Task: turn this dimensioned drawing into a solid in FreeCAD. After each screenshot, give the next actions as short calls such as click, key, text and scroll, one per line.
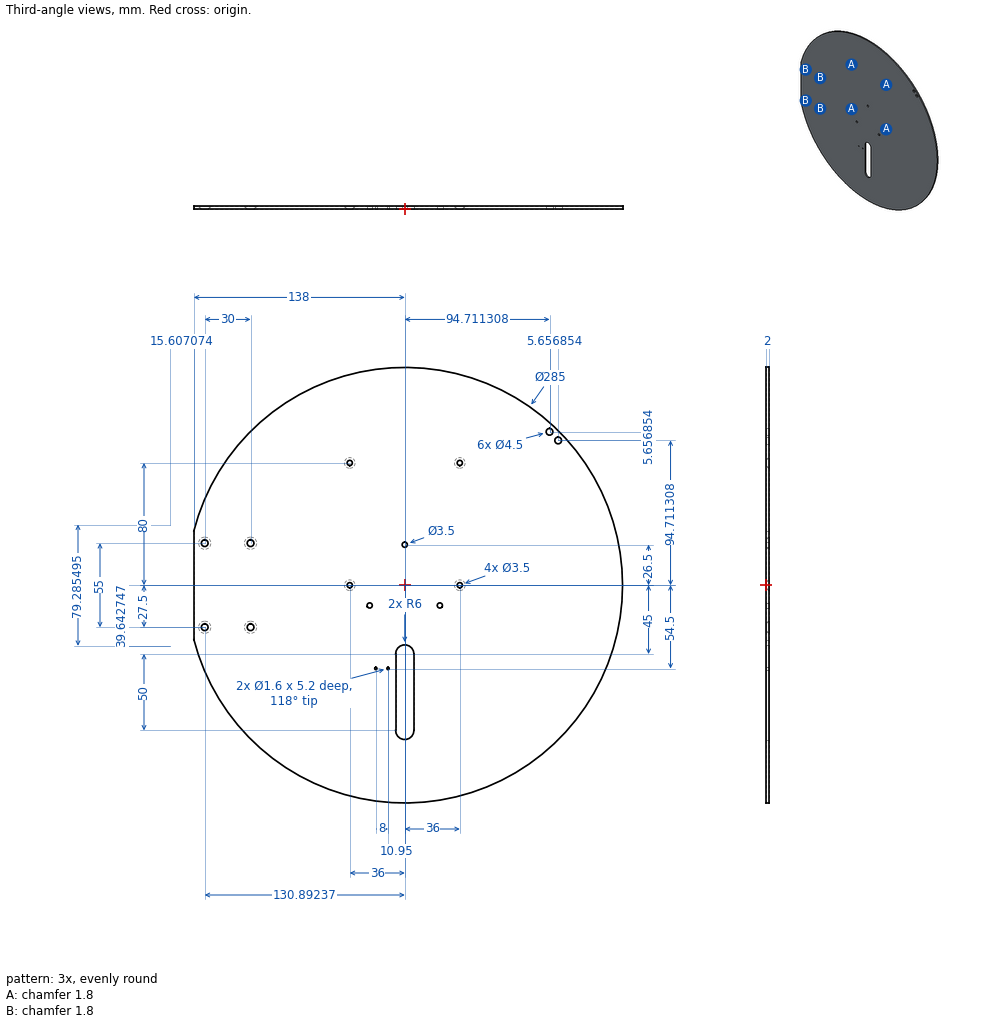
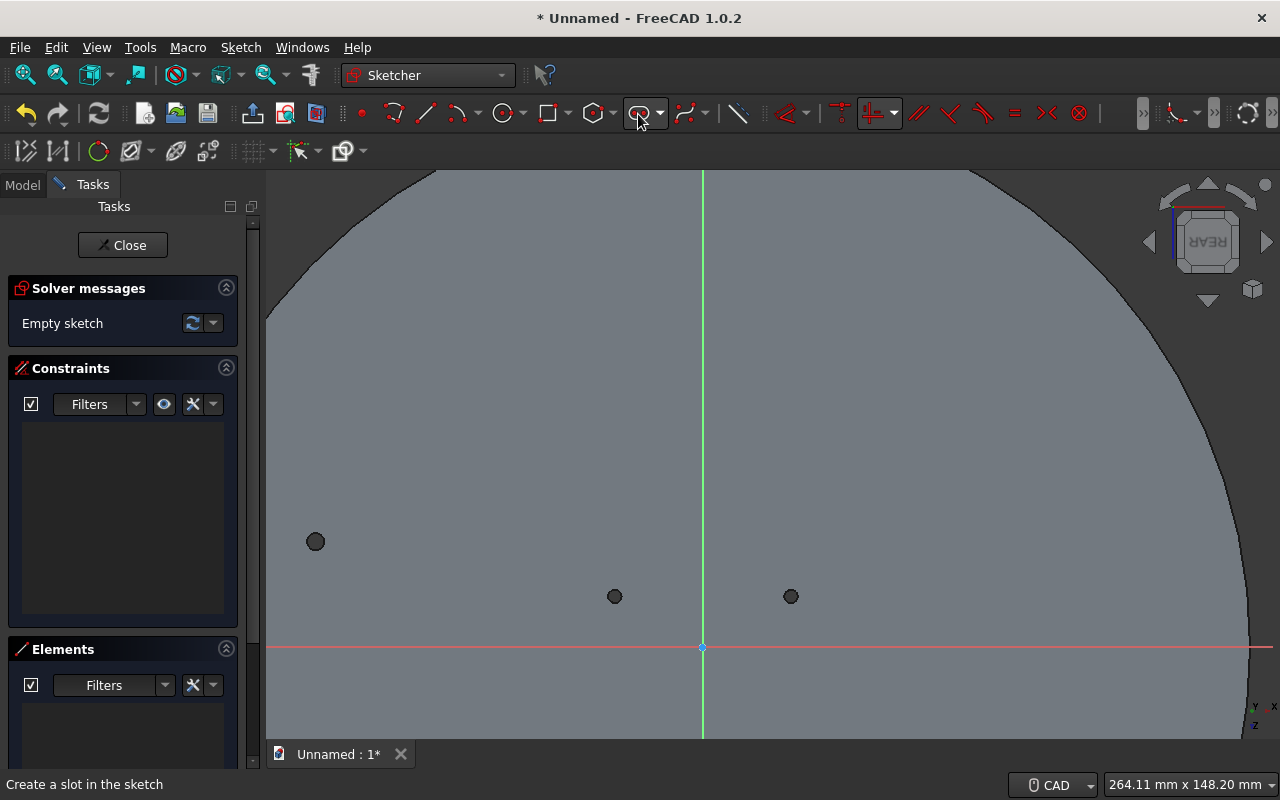
click(703, 475)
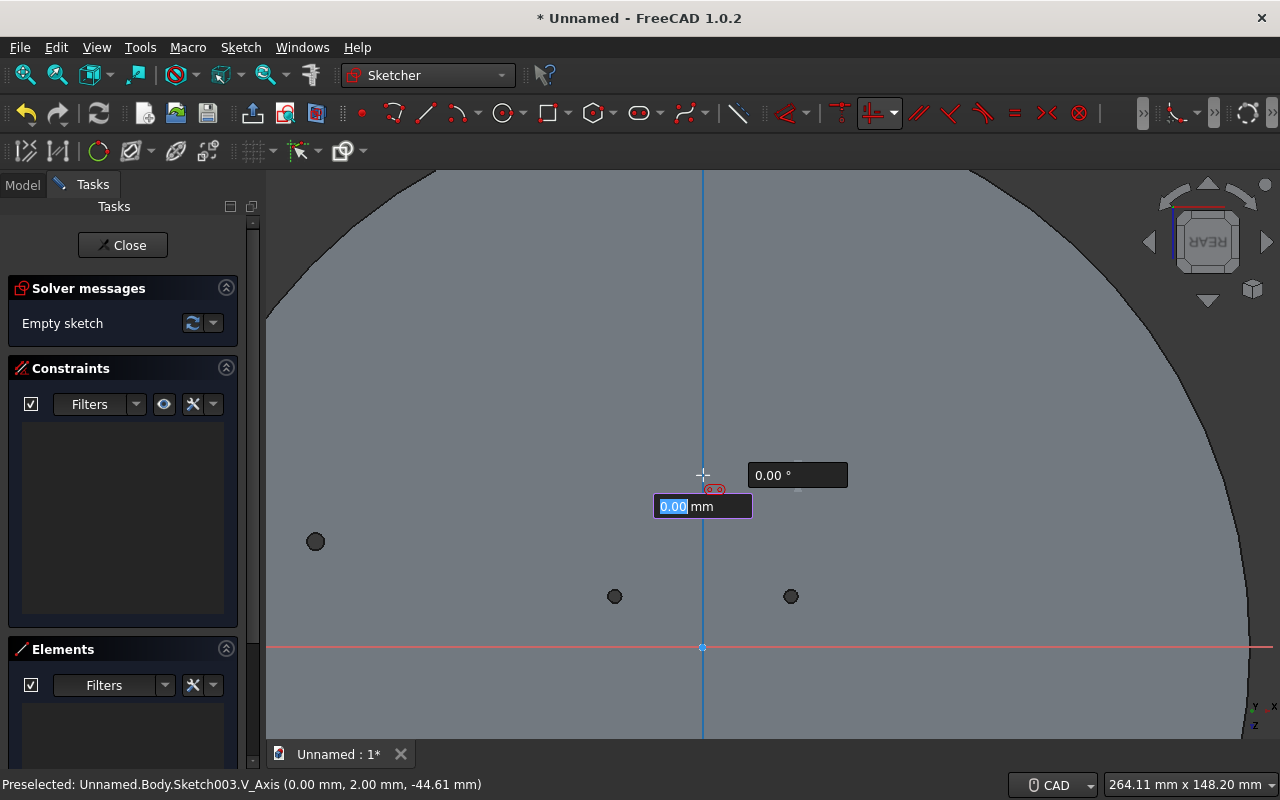
click(712, 283)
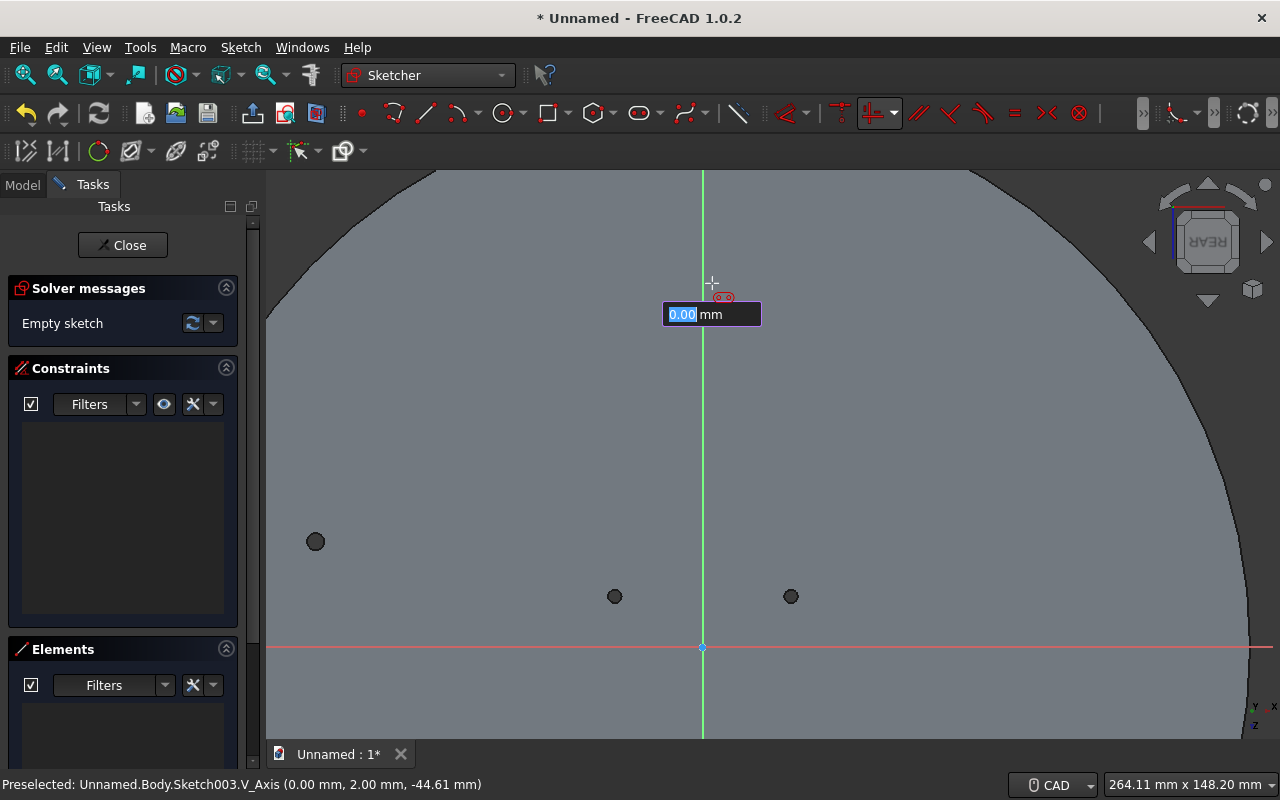
click(680, 379)
key(Escape)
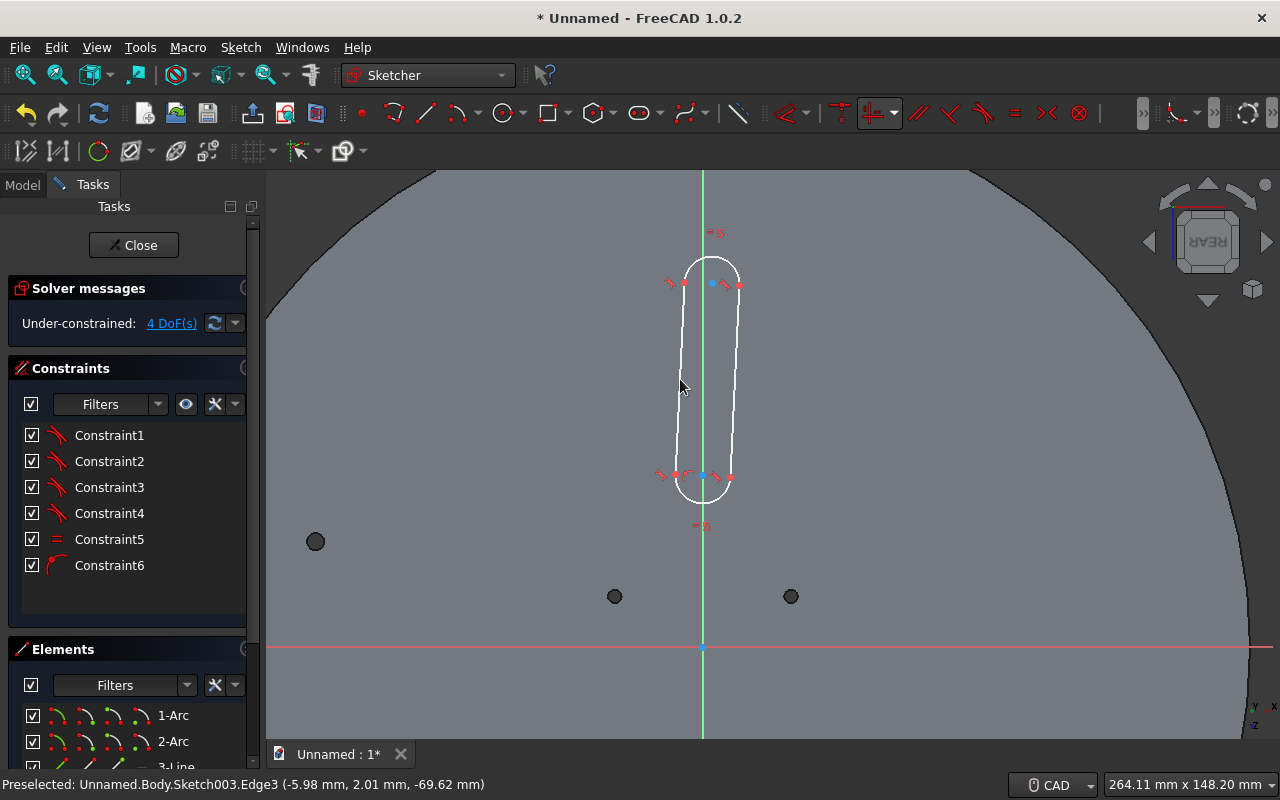
click(678, 417)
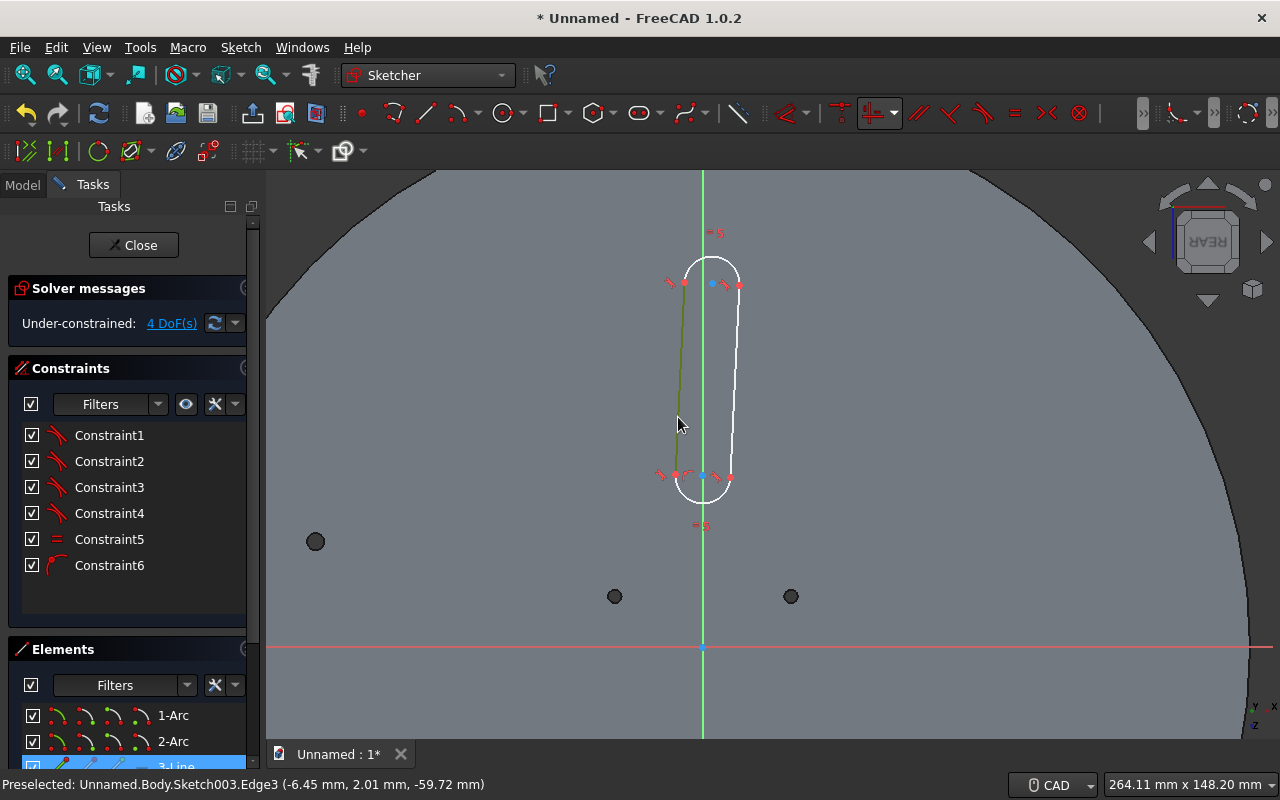
click(896, 114)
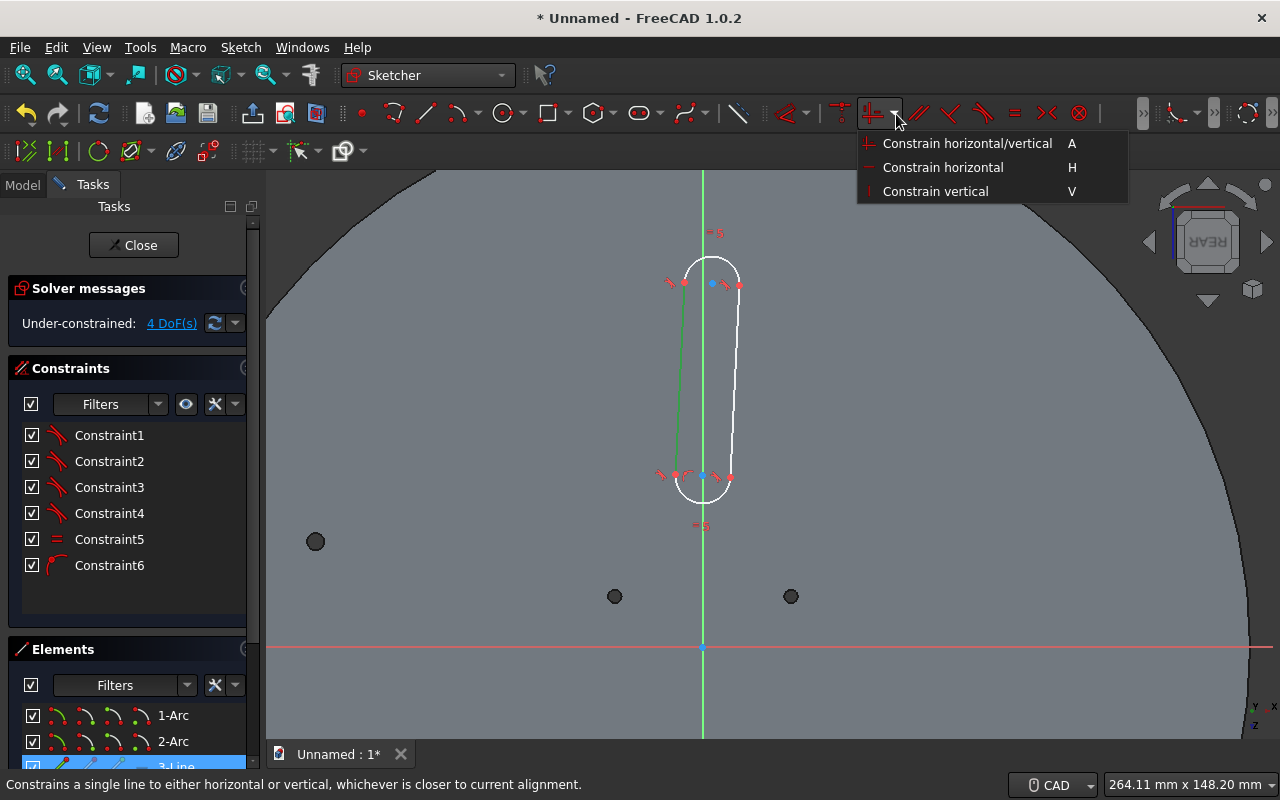
click(993, 191)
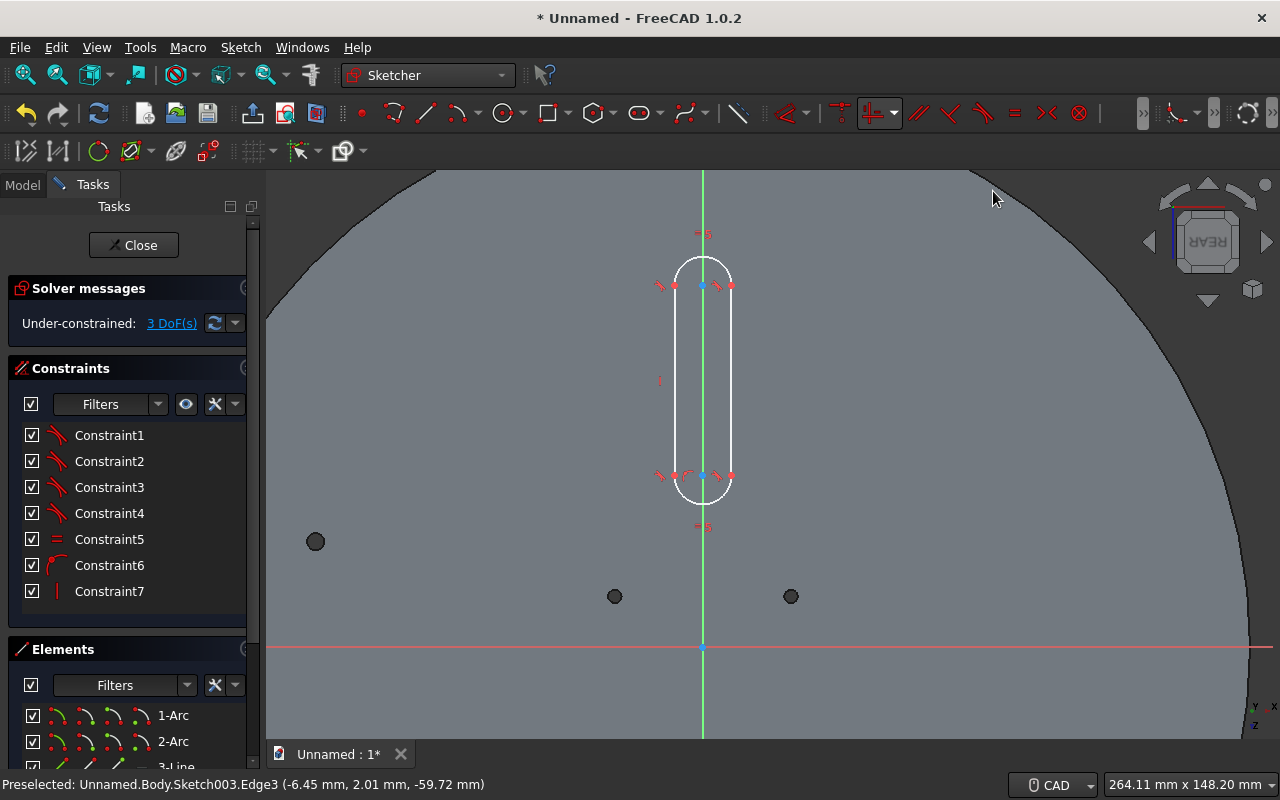
click(786, 114)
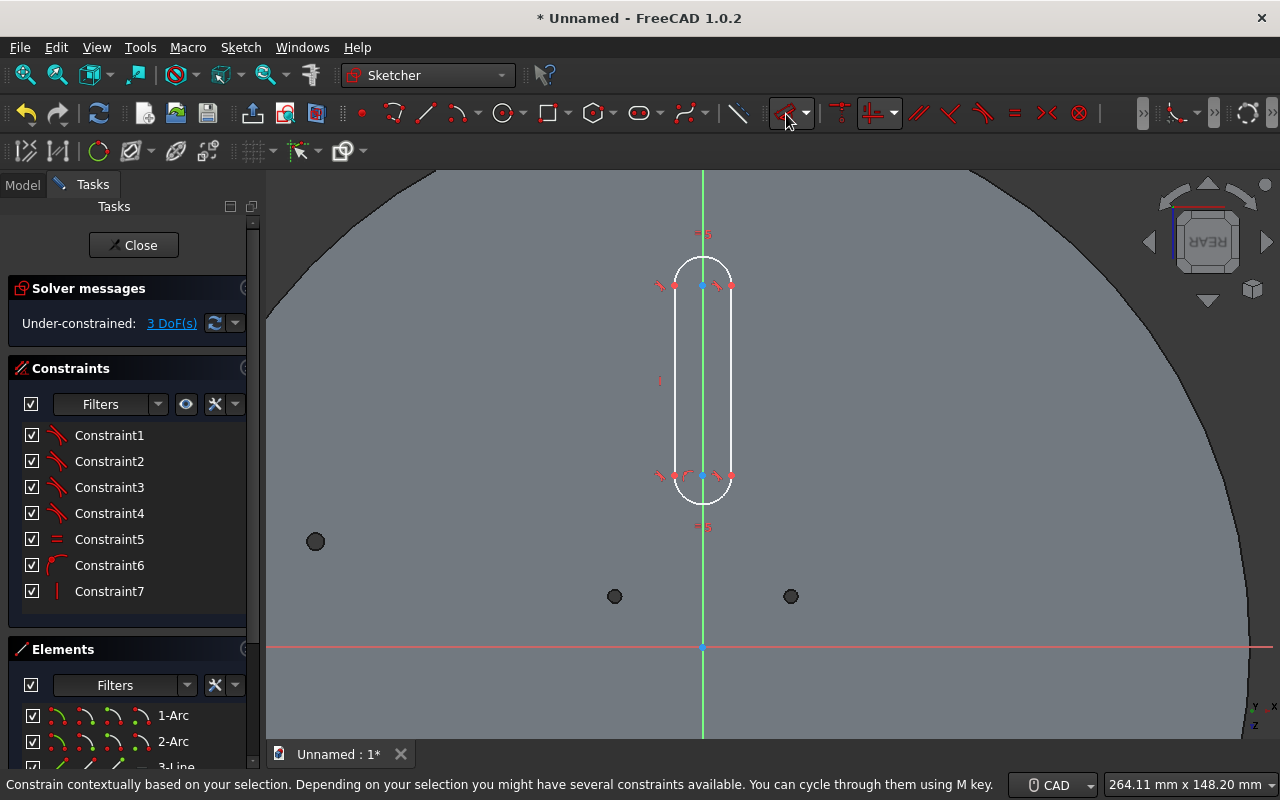
scroll(686, 499, up, 3)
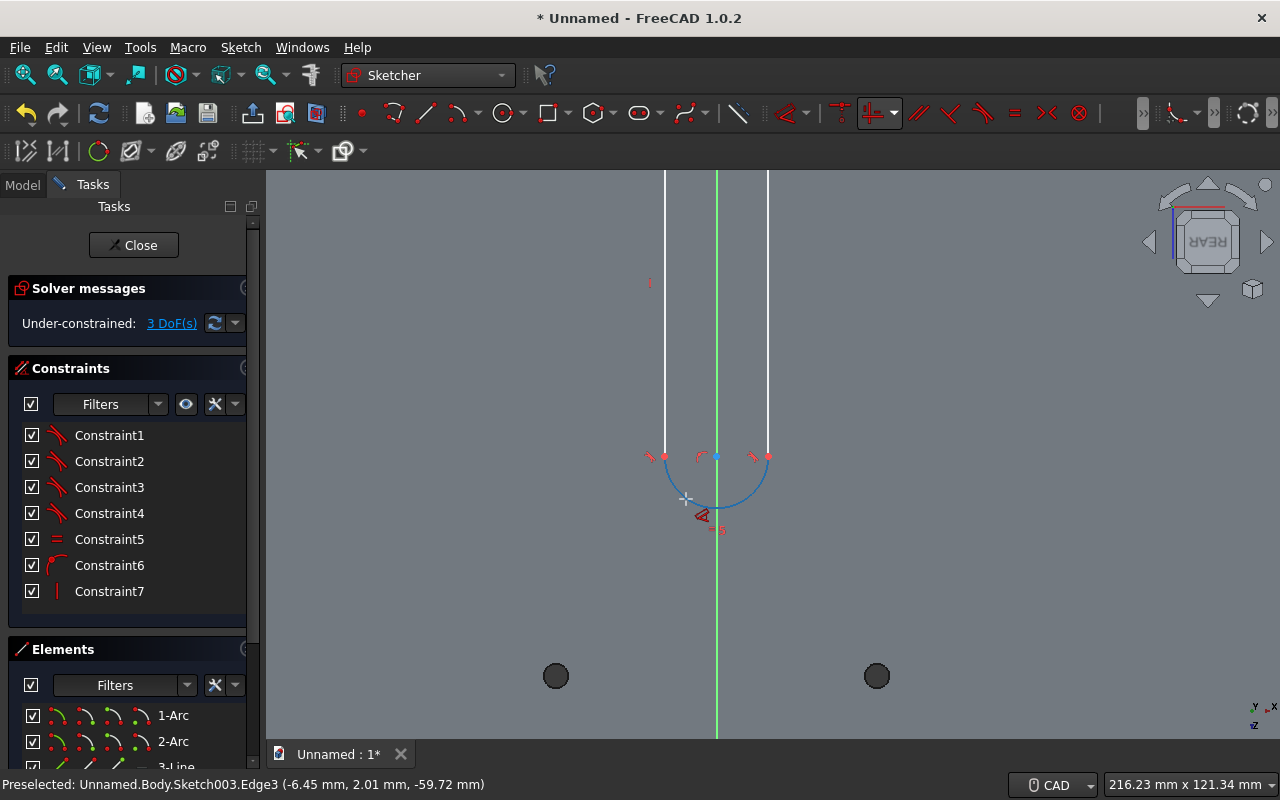
click(686, 498)
click(667, 524)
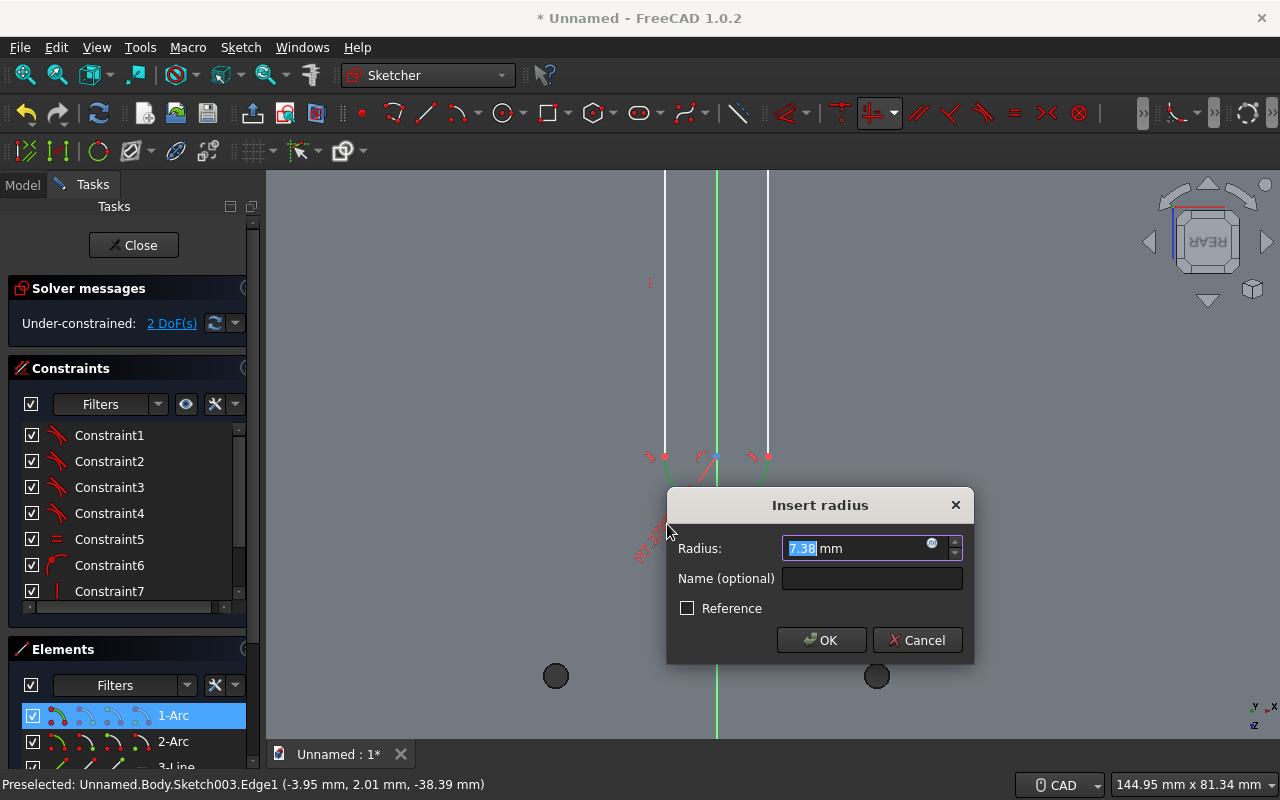
text(6)
key(Return)